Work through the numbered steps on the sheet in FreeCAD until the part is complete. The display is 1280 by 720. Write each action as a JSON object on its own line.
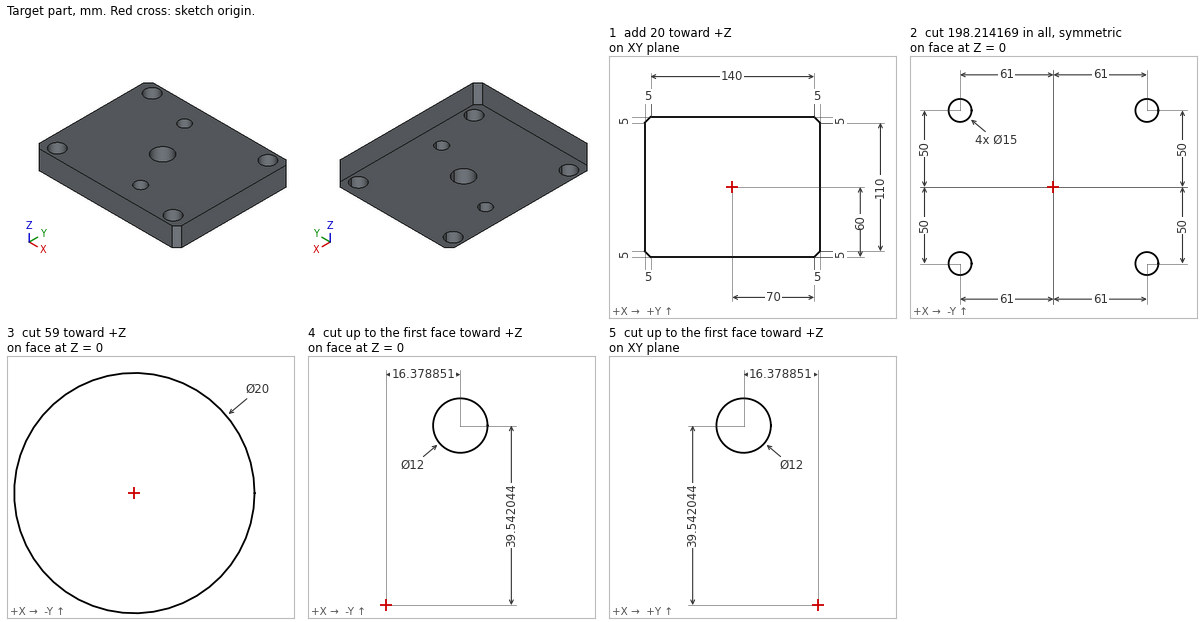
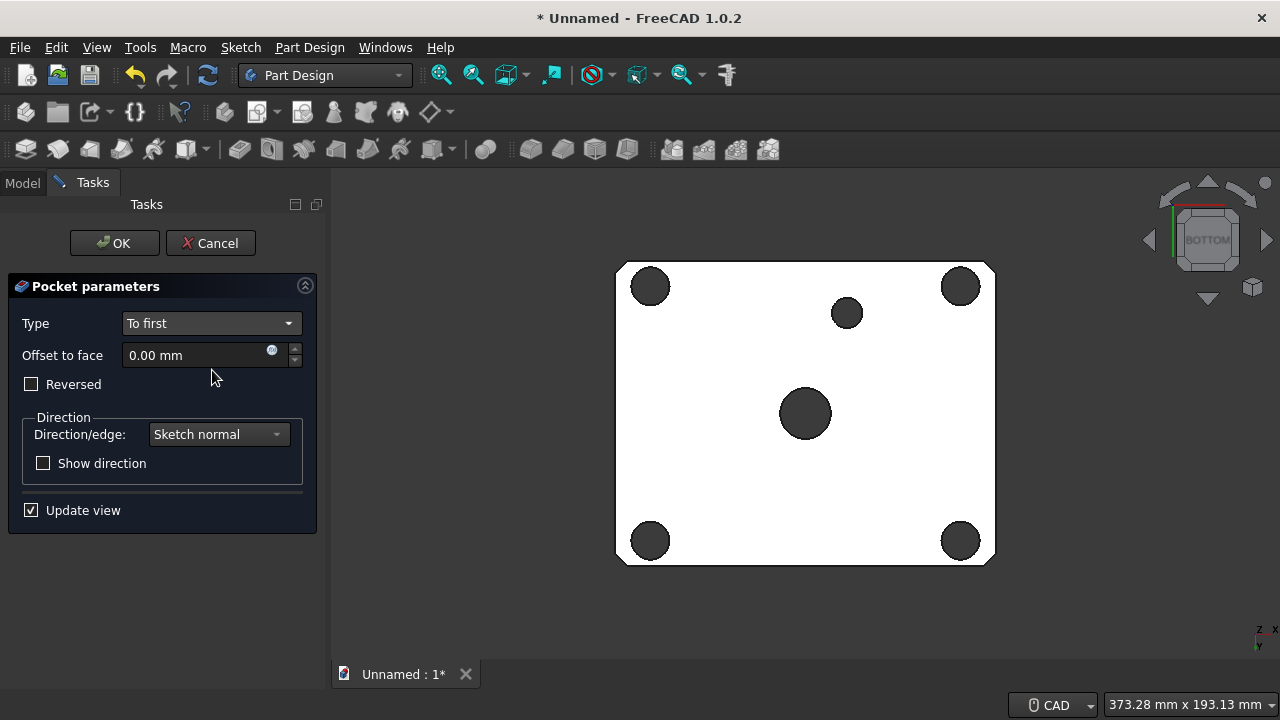
{"action": "left_click", "coordinate": [115, 243]}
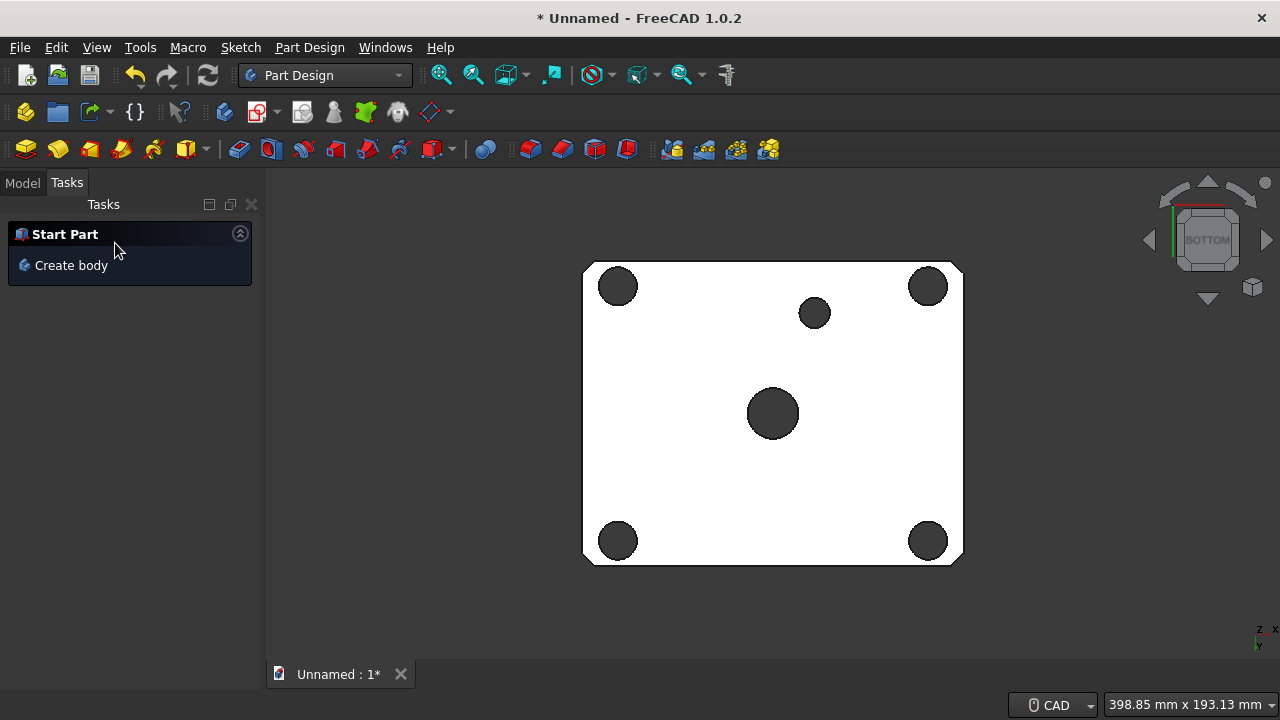
{"action": "left_click", "coordinate": [258, 112]}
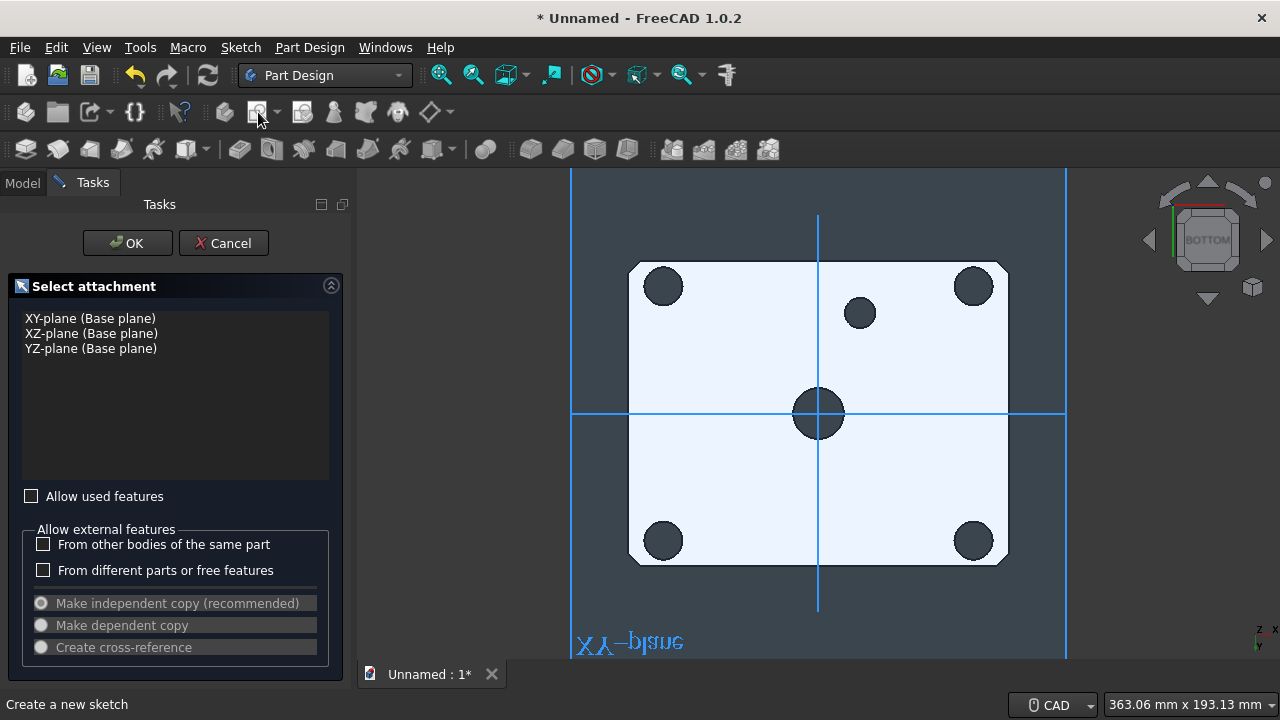
{"action": "left_click", "coordinate": [82, 318]}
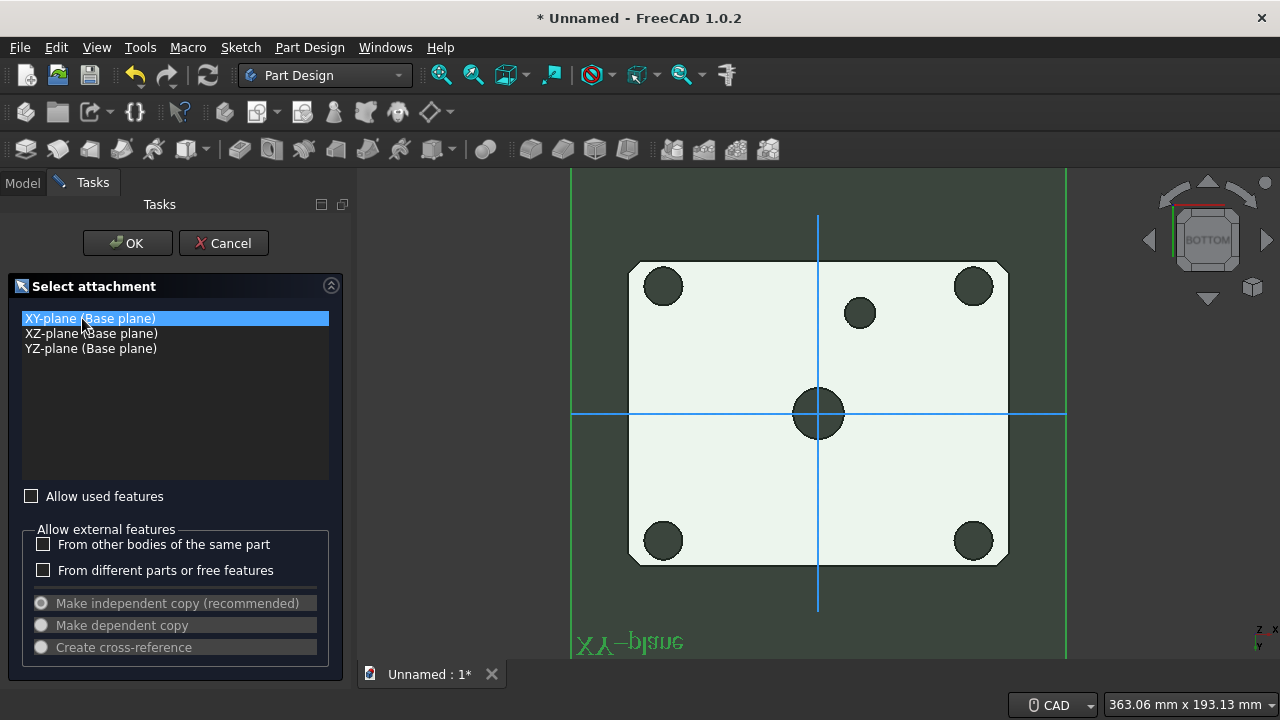
{"action": "left_click", "coordinate": [128, 243]}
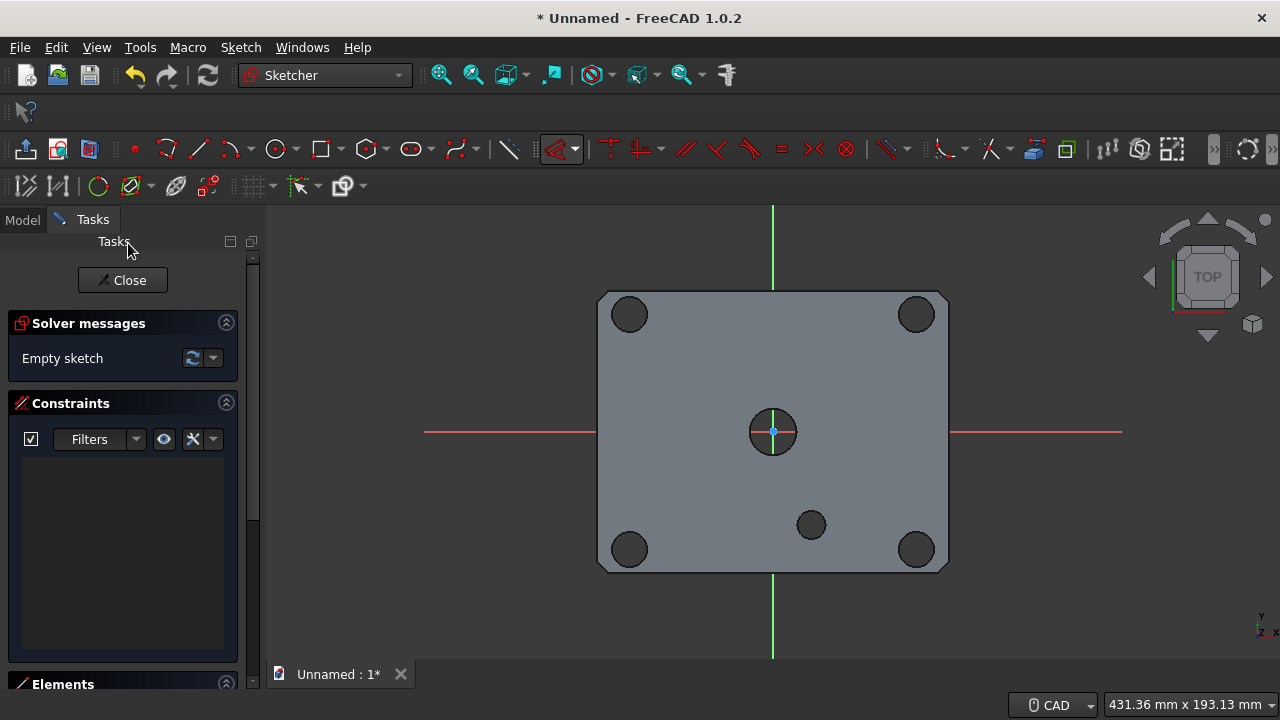
{"action": "key", "text": "q s"}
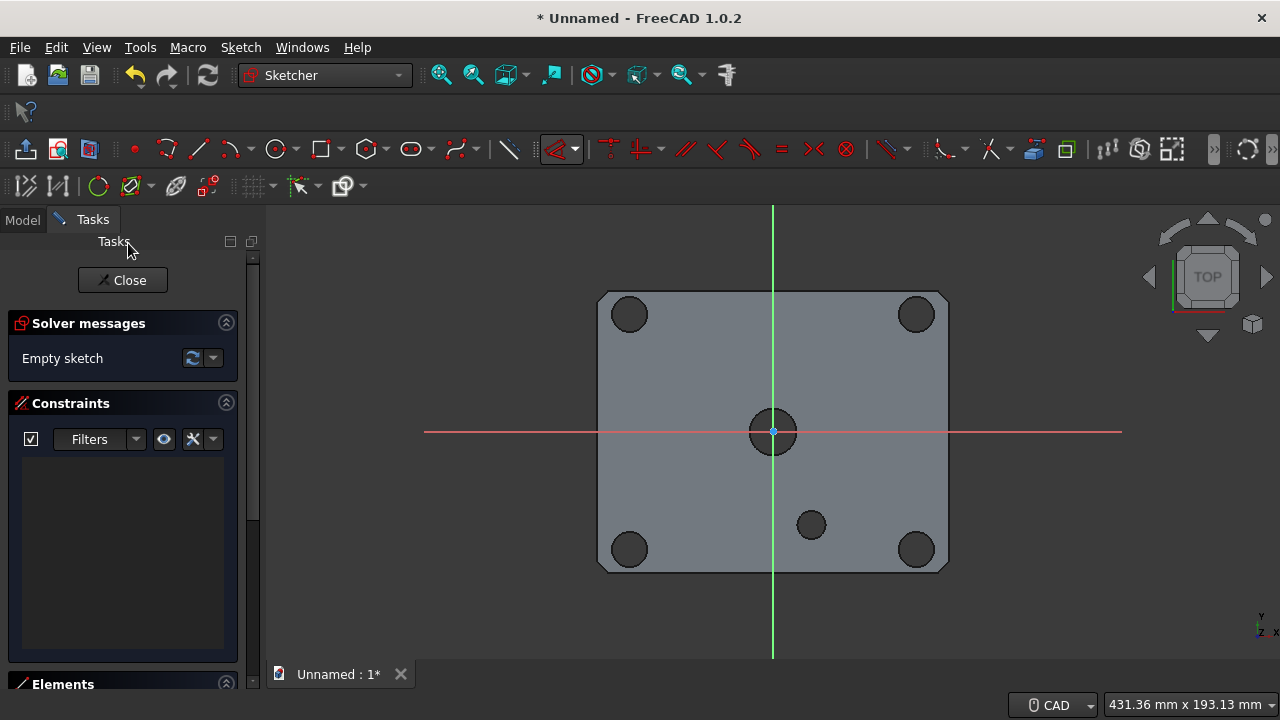
{"action": "scroll", "coordinate": [738, 327], "scroll_direction": "up", "scroll_amount": 11}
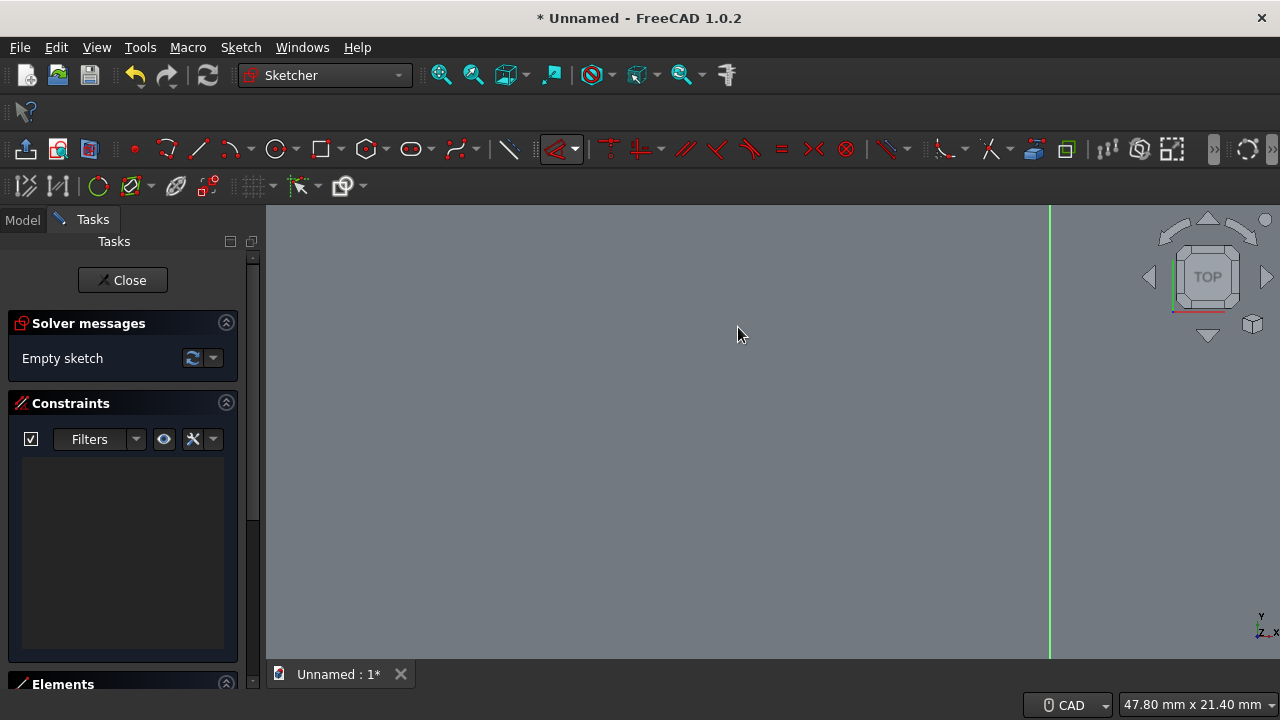
{"action": "key", "text": "g c"}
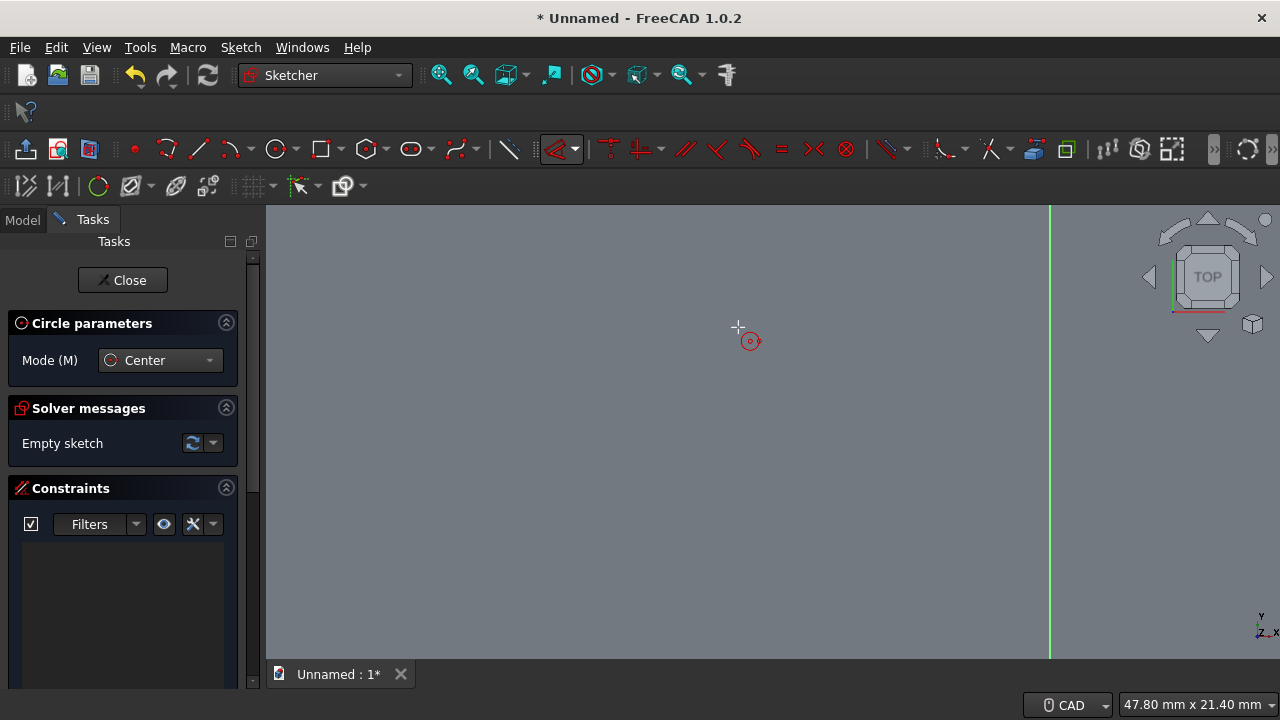
{"action": "left_click", "coordinate": [703, 434]}
{"action": "mouse_move", "coordinate": [793, 344]}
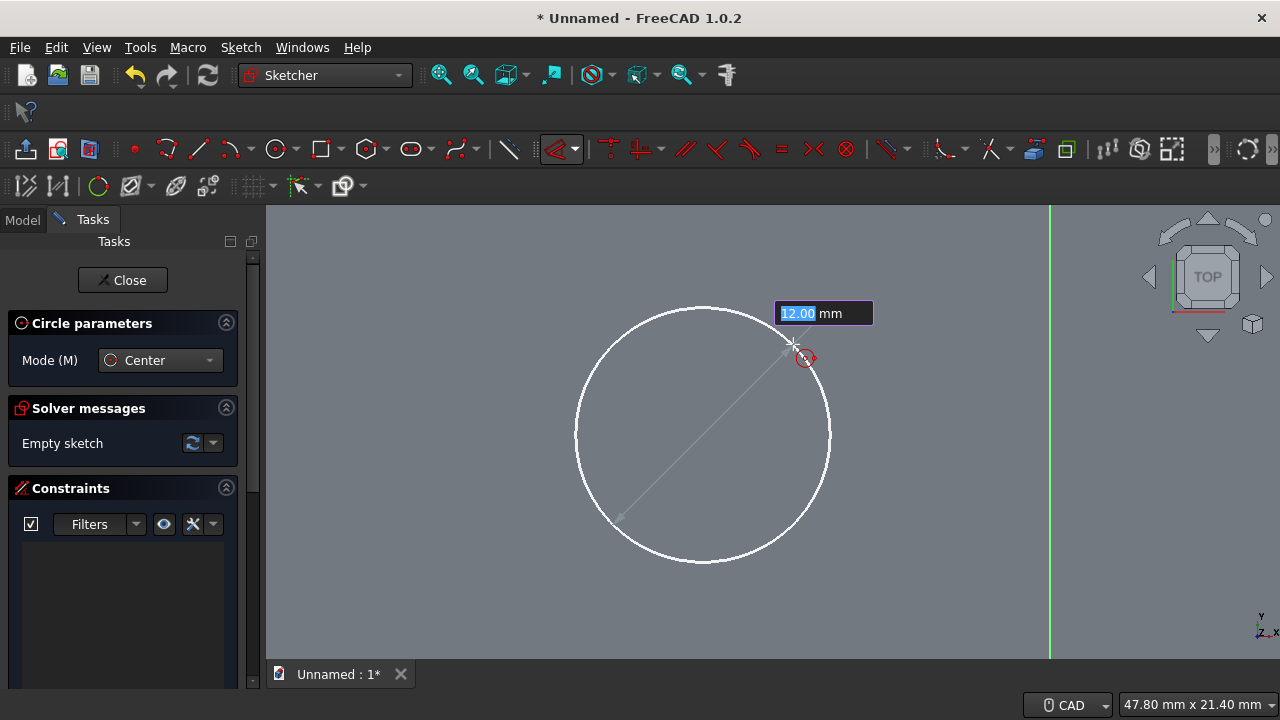
{"action": "type", "text": "12"}
{"action": "key", "text": "Return"}
{"action": "key", "text": "Escape"}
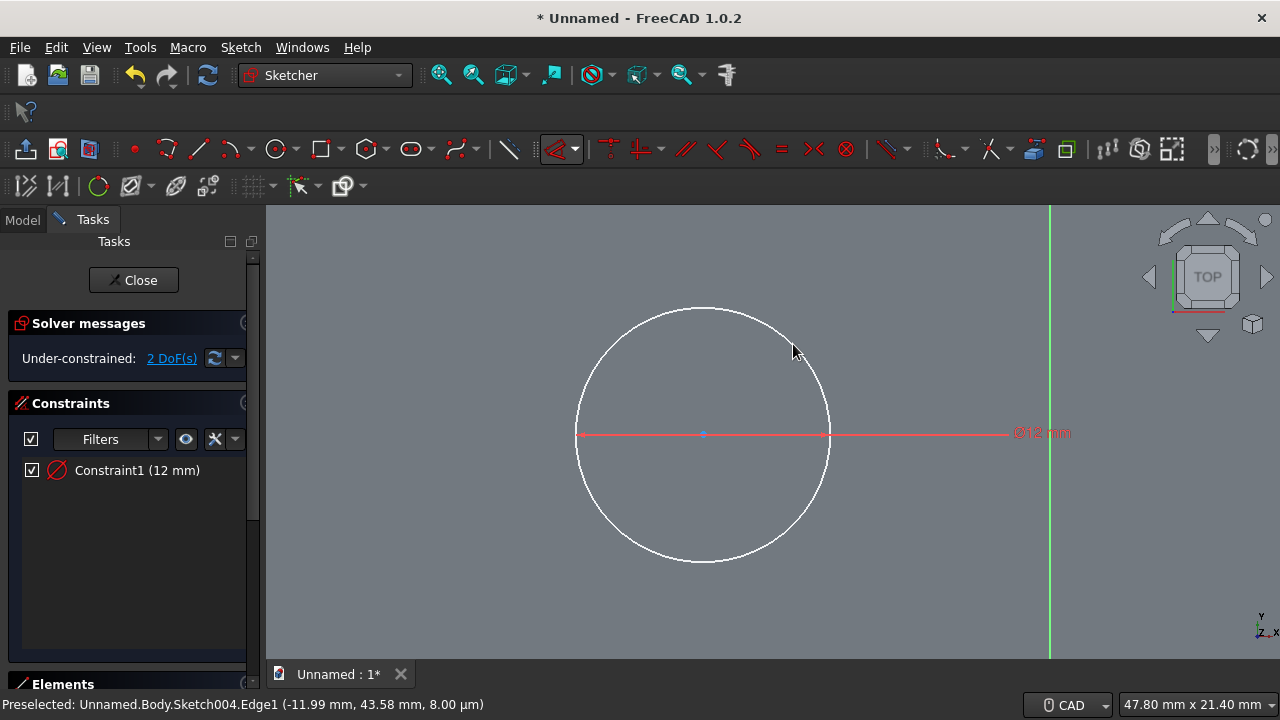
{"action": "left_click", "coordinate": [703, 435]}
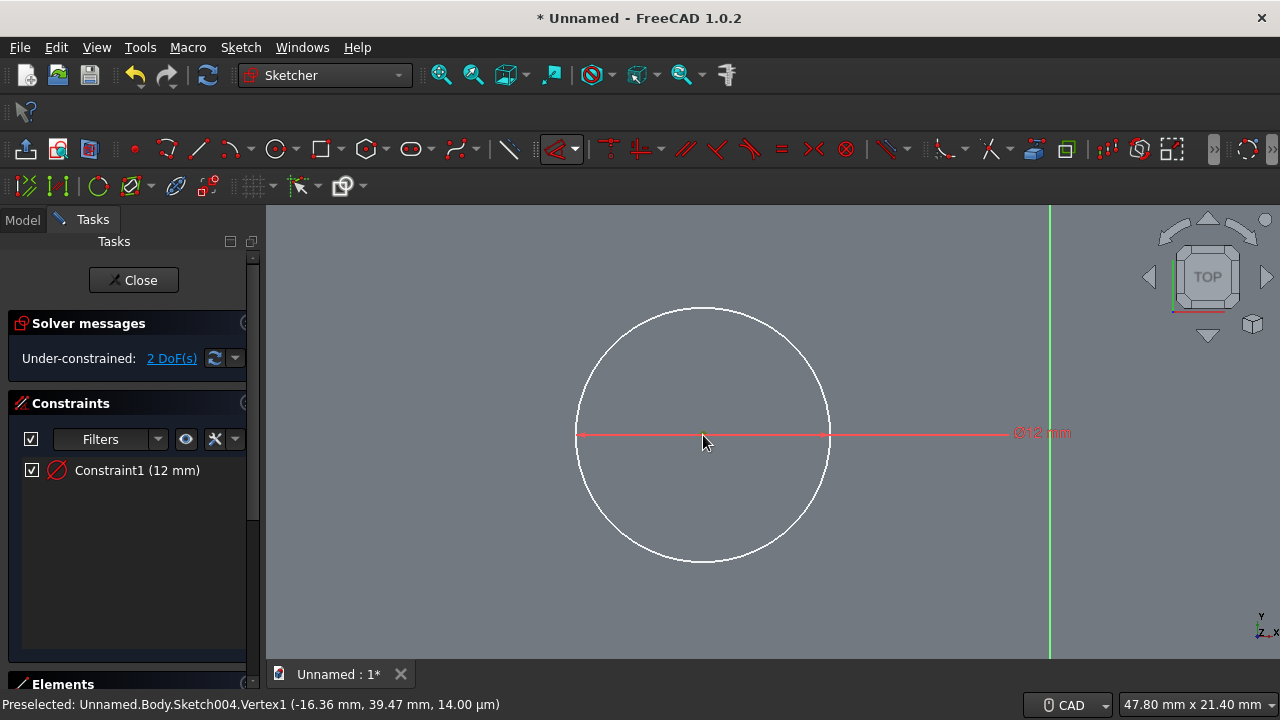
{"action": "key", "text": "l"}